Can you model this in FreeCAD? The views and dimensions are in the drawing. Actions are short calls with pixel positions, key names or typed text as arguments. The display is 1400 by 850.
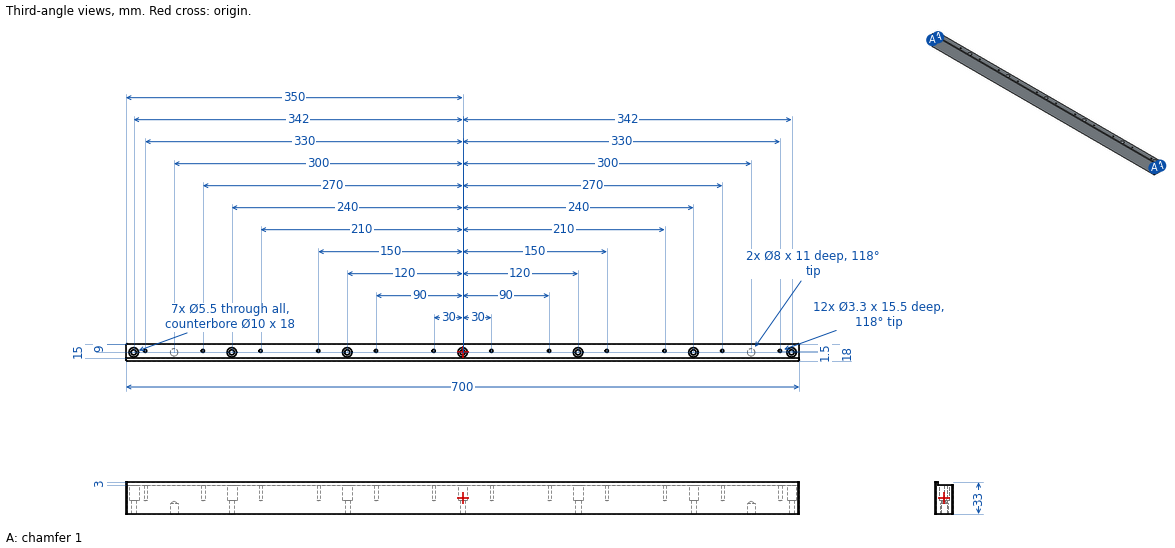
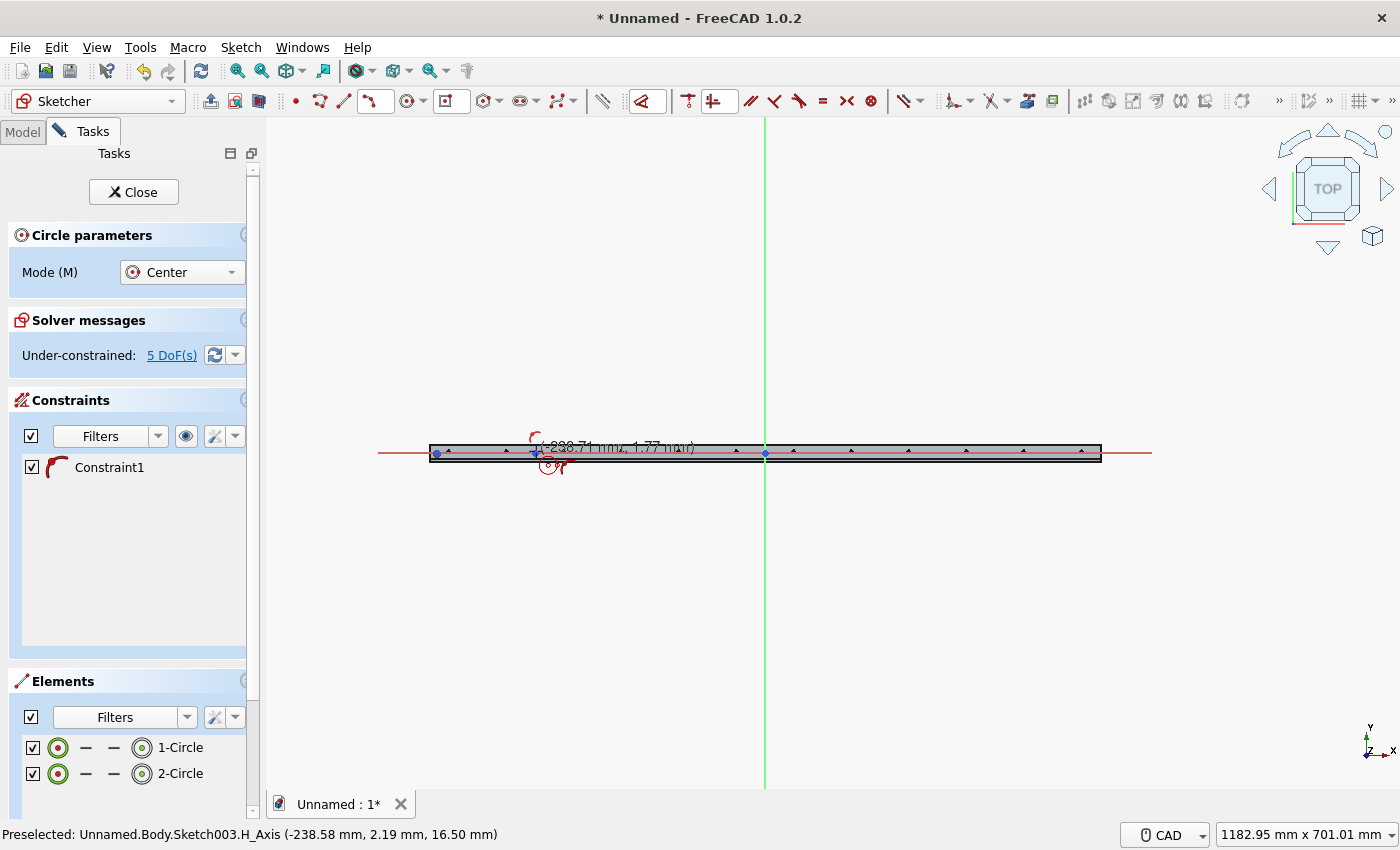
scroll(650, 453, up, 11)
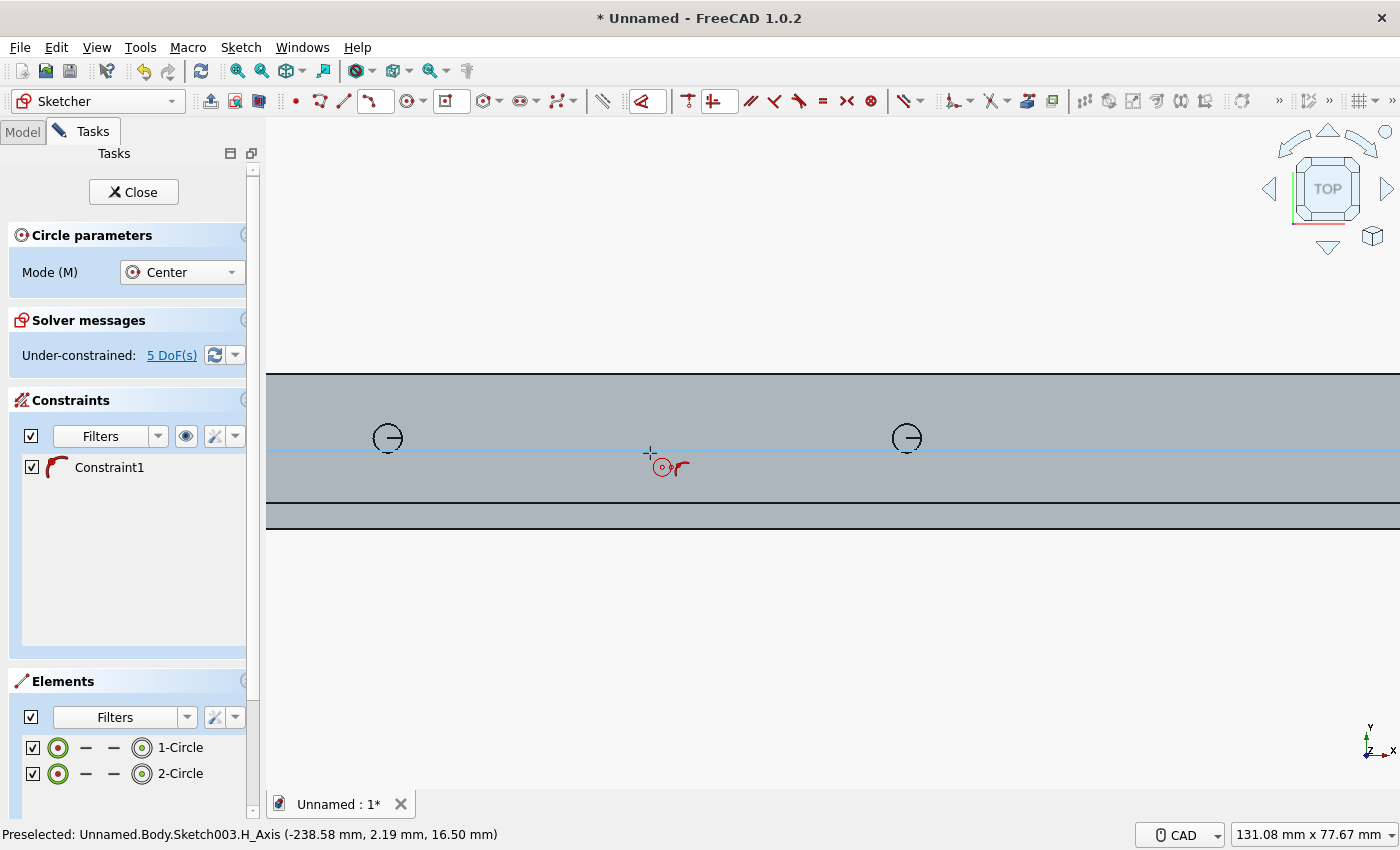
scroll(650, 453, down, 11)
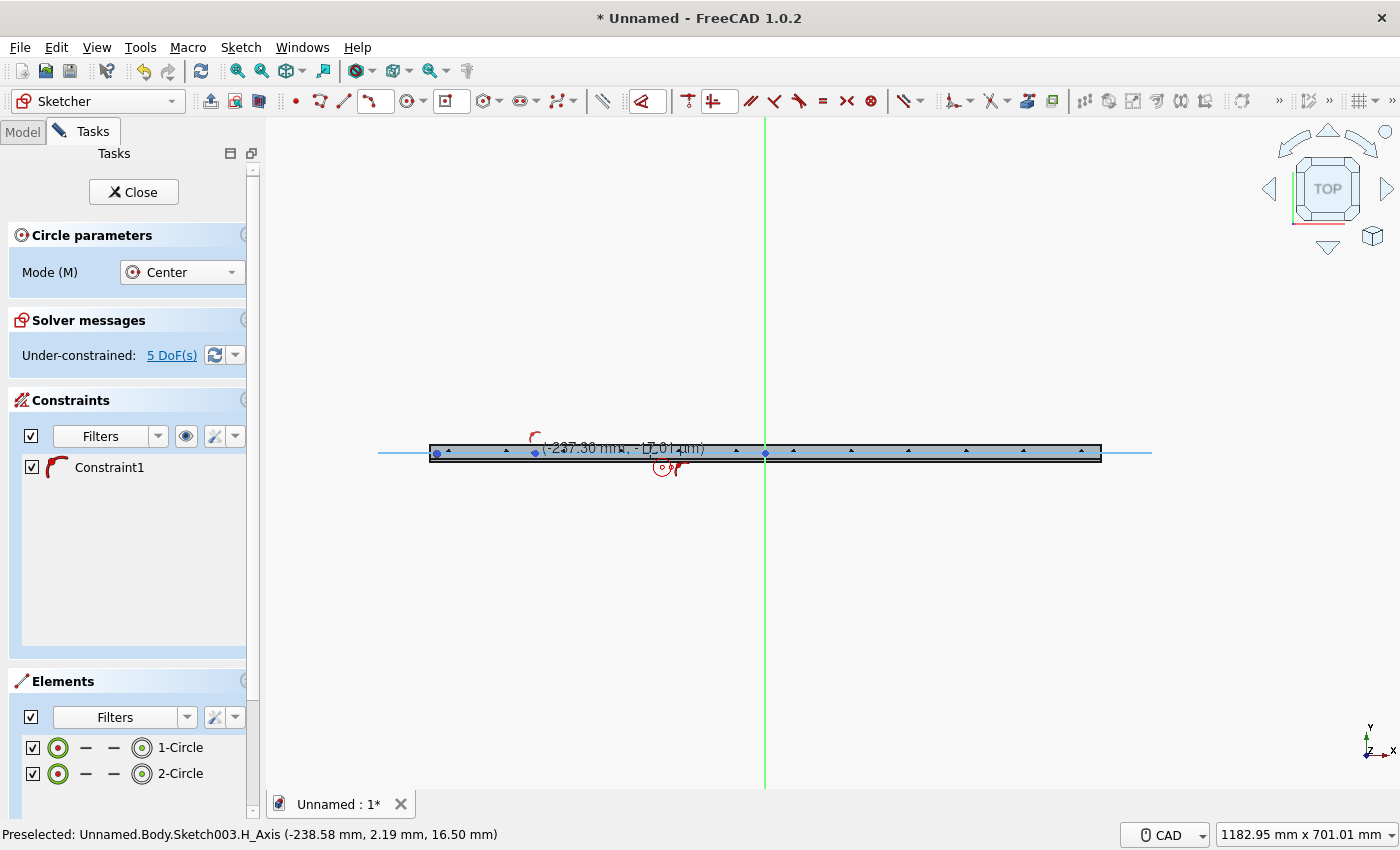
click(650, 453)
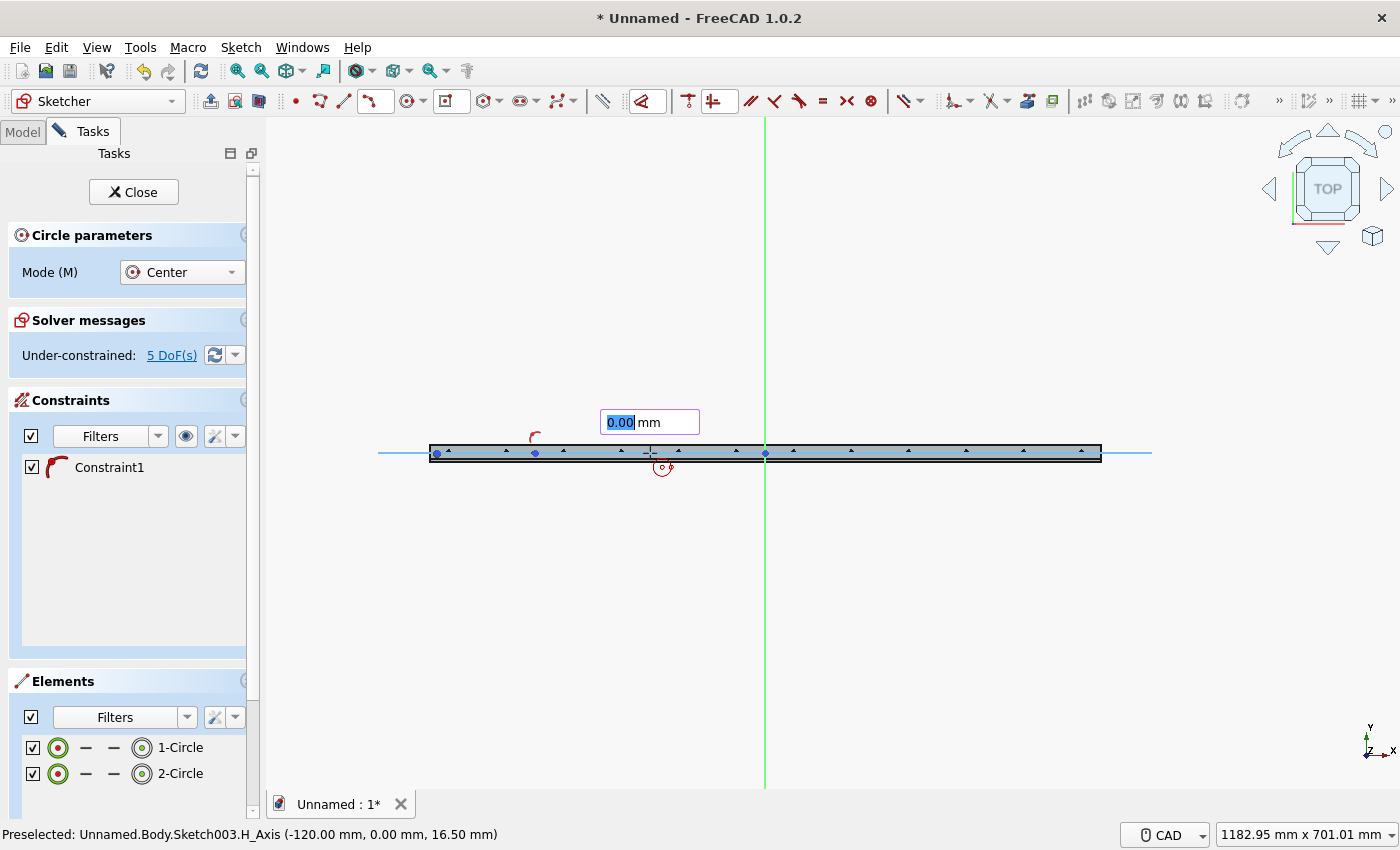
scroll(651, 451, up, 10)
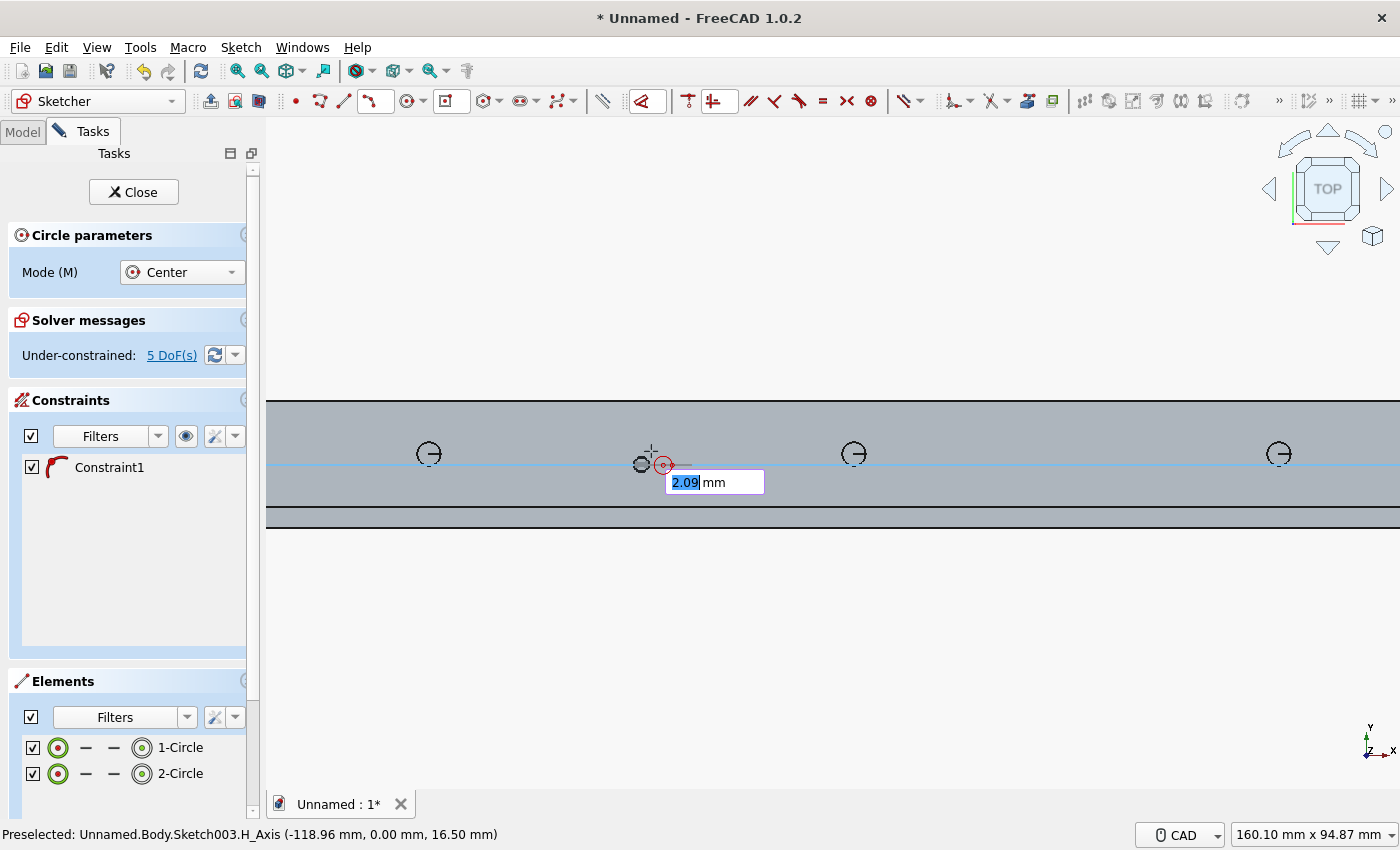
click(648, 446)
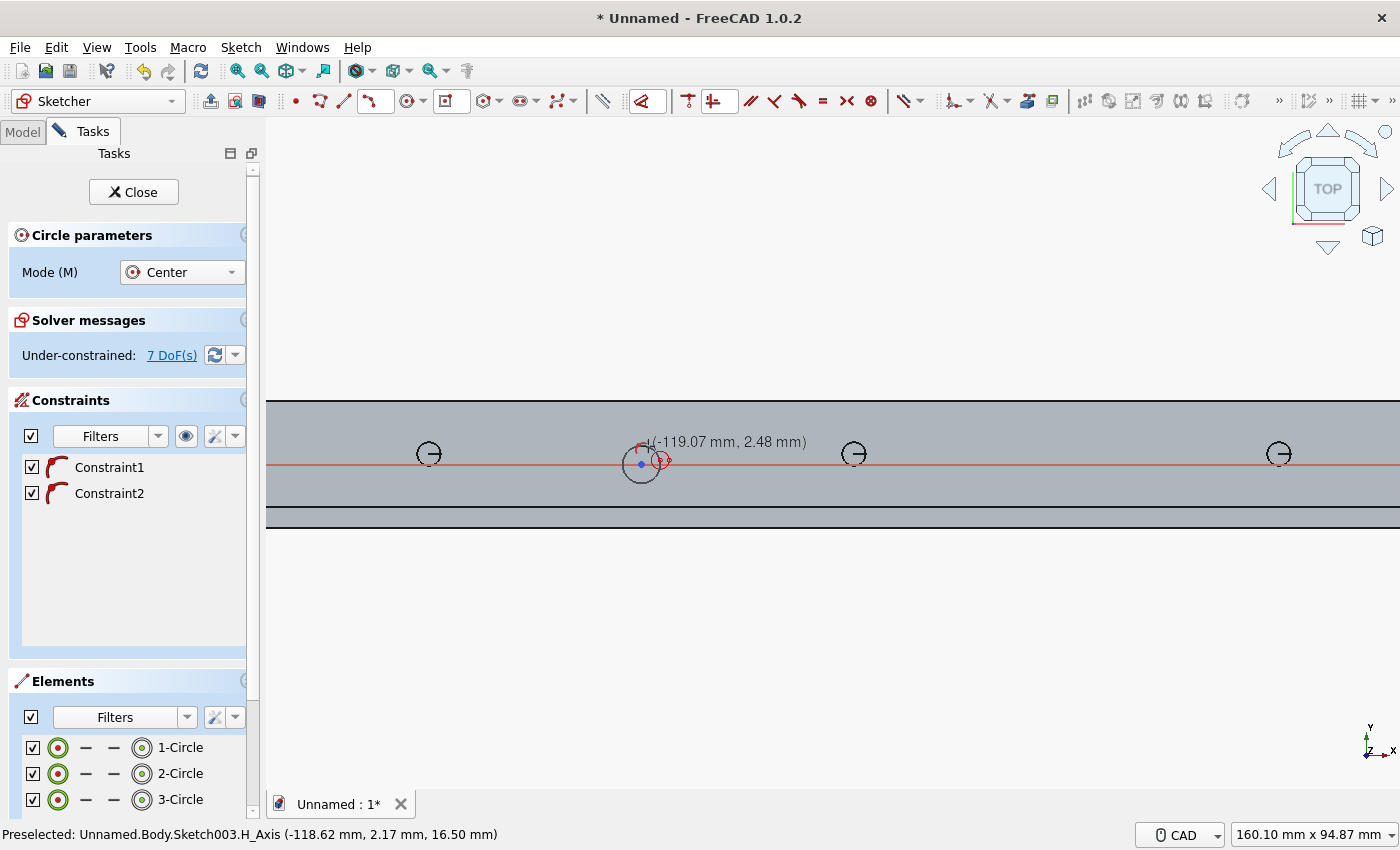
scroll(651, 451, down, 10)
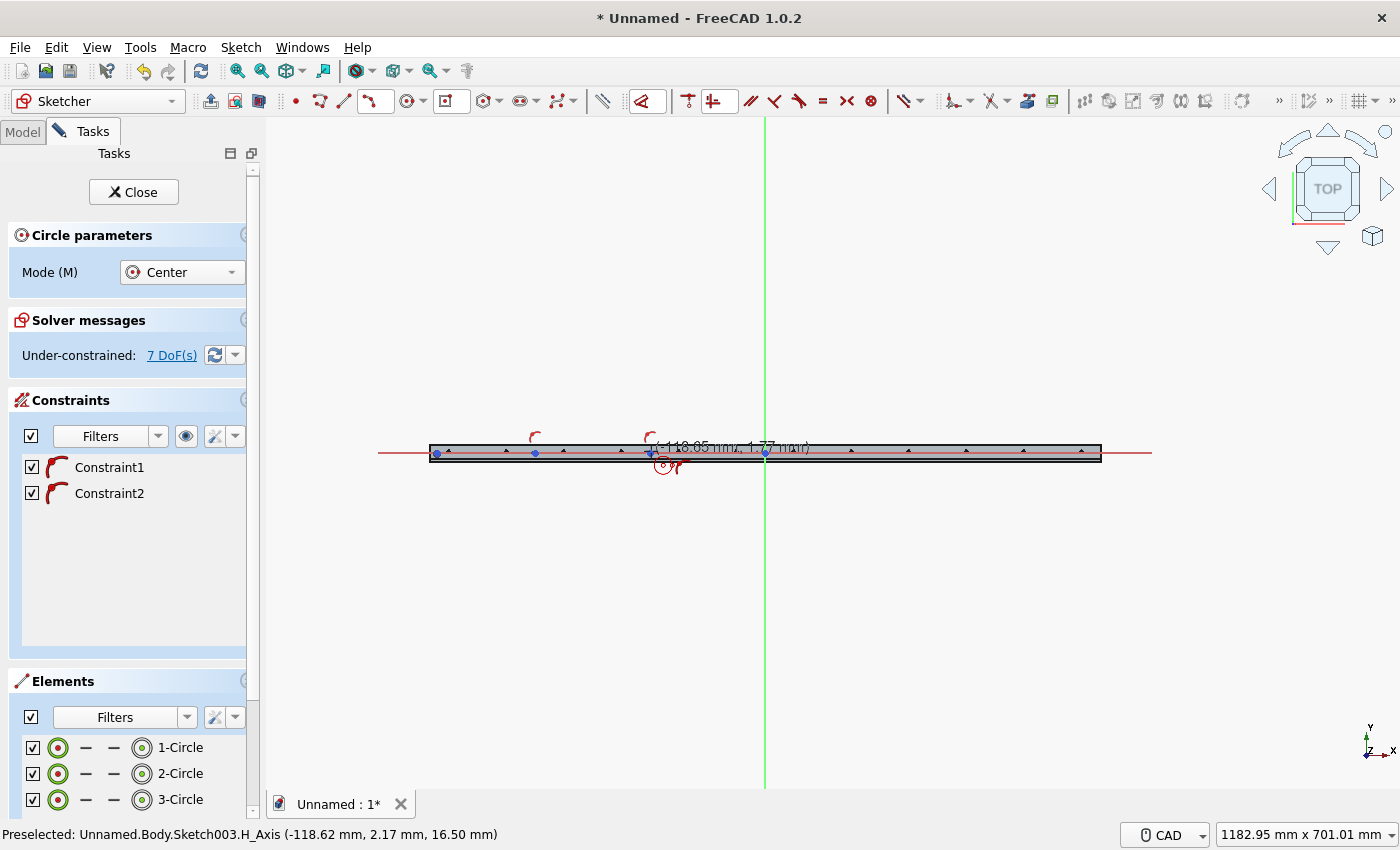
scroll(765, 453, up, 11)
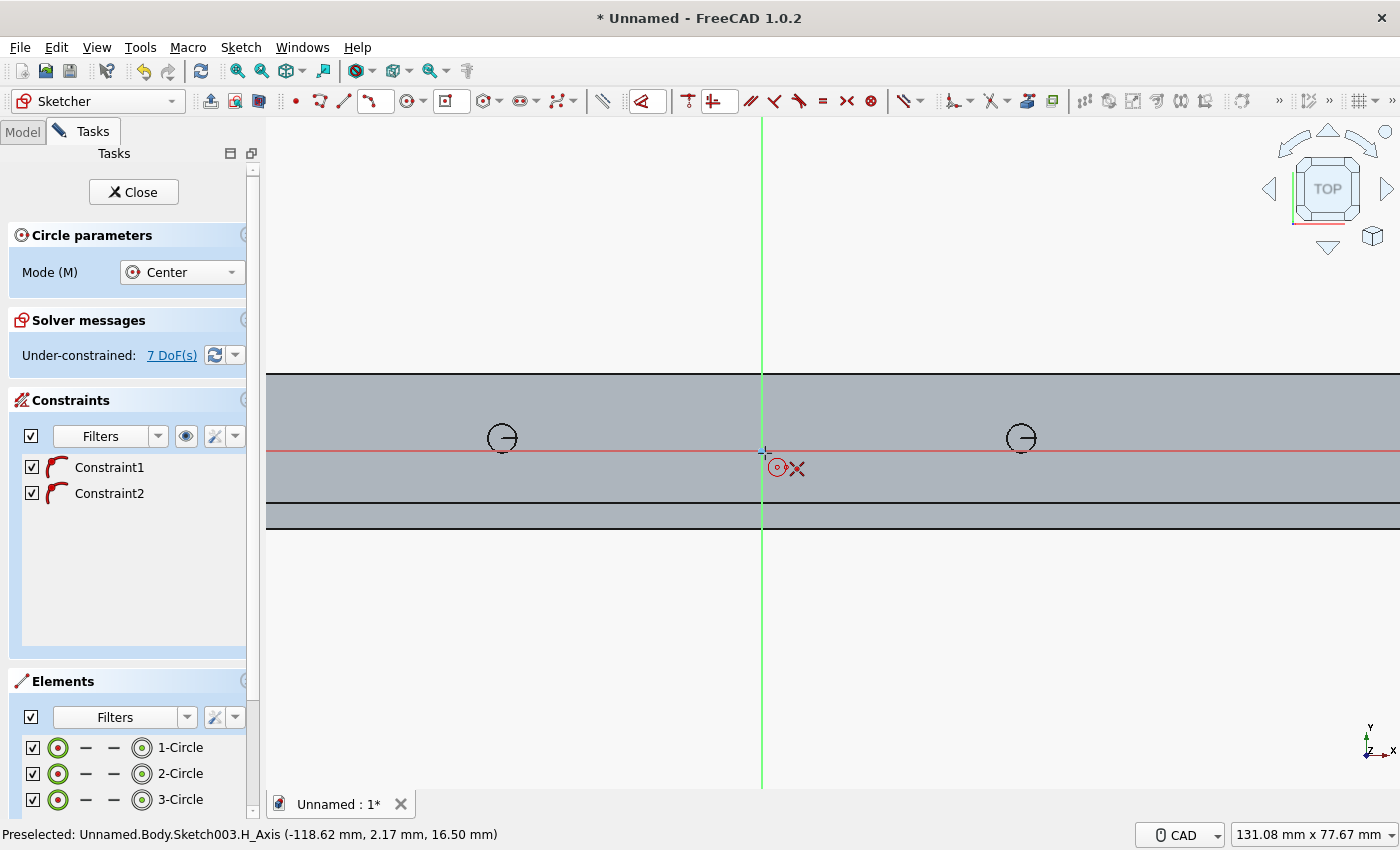
scroll(765, 453, down, 11)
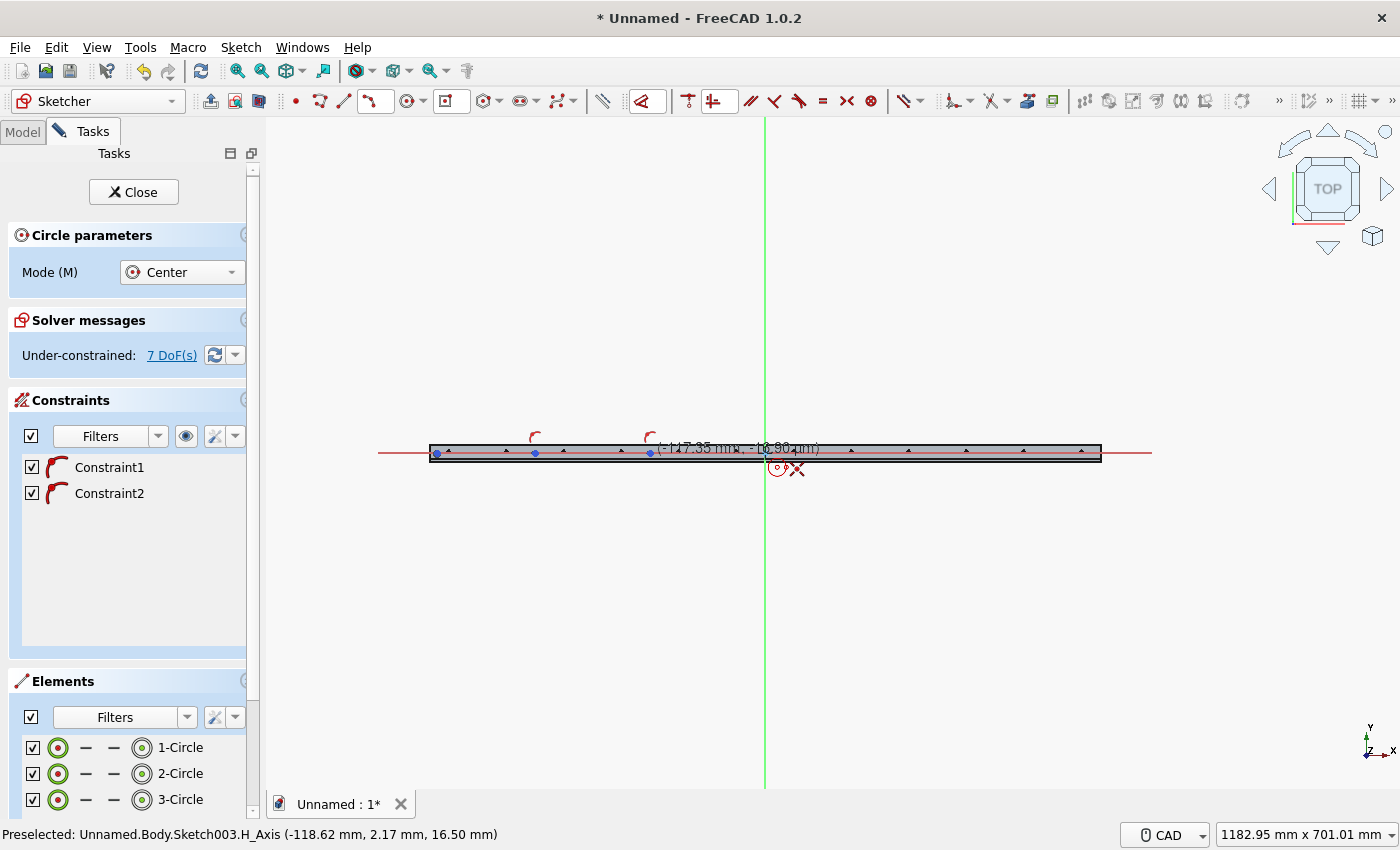
click(765, 453)